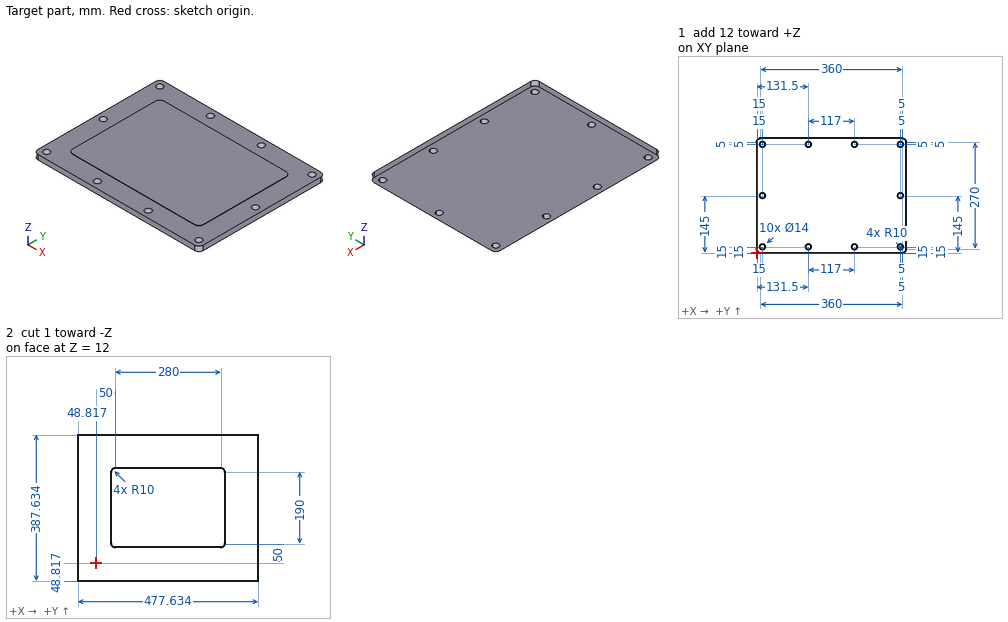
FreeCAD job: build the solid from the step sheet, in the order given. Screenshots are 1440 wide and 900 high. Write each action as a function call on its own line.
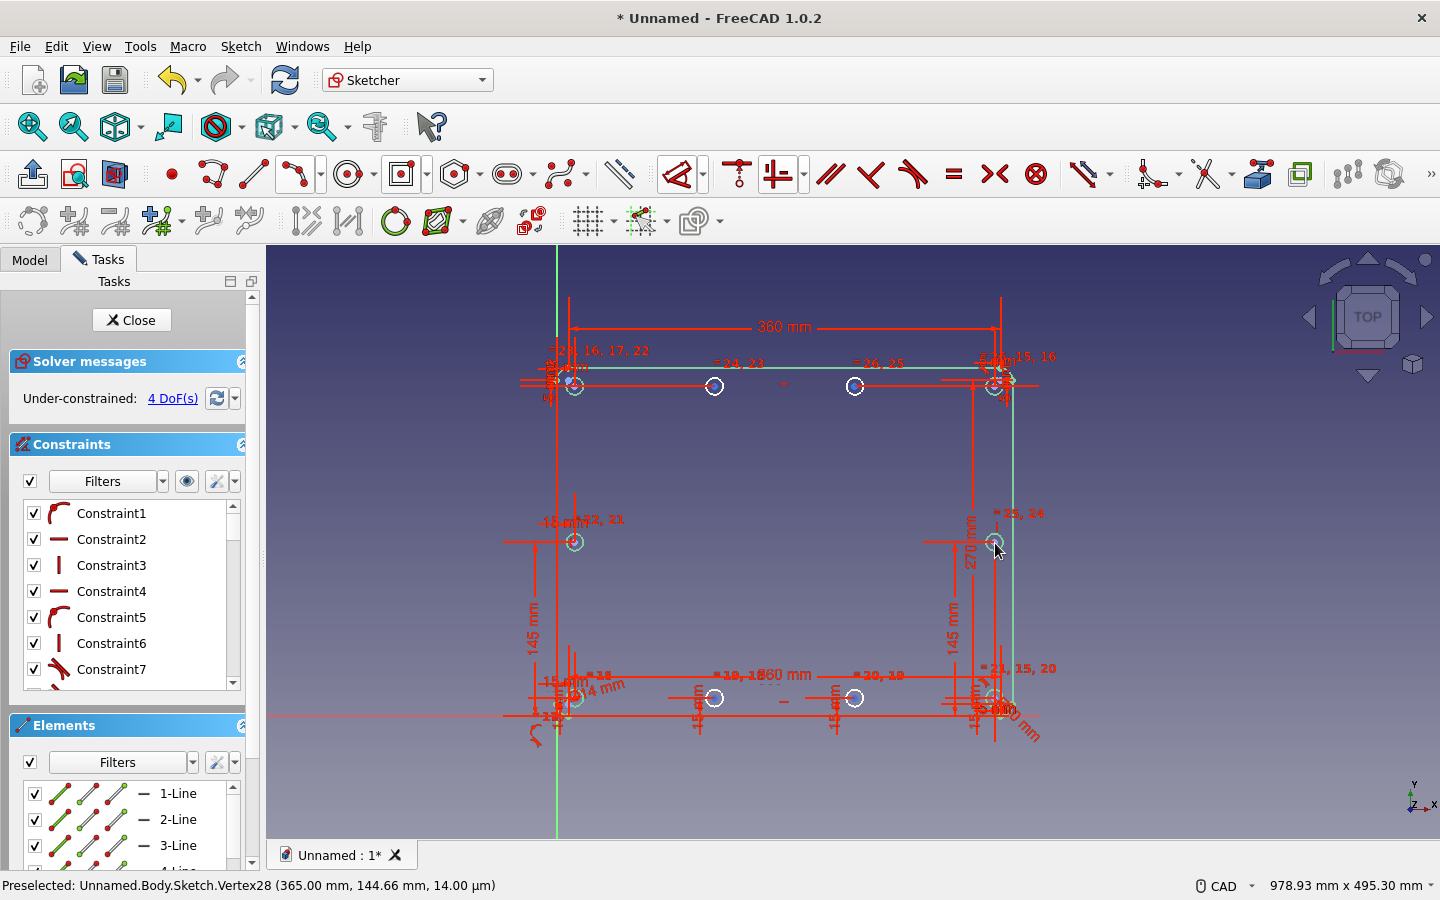
click(715, 698)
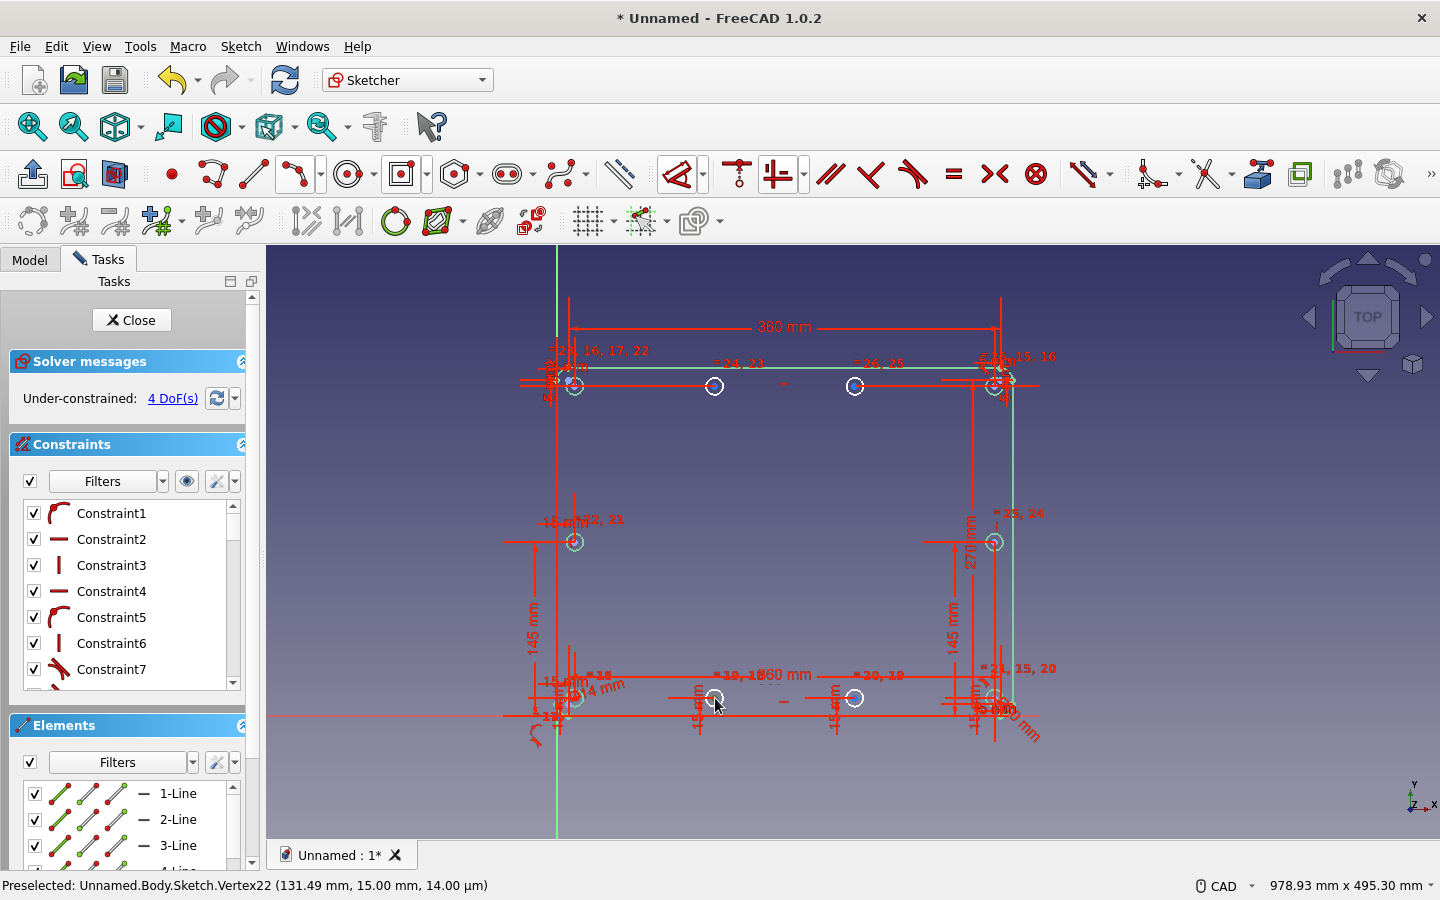
click(855, 698)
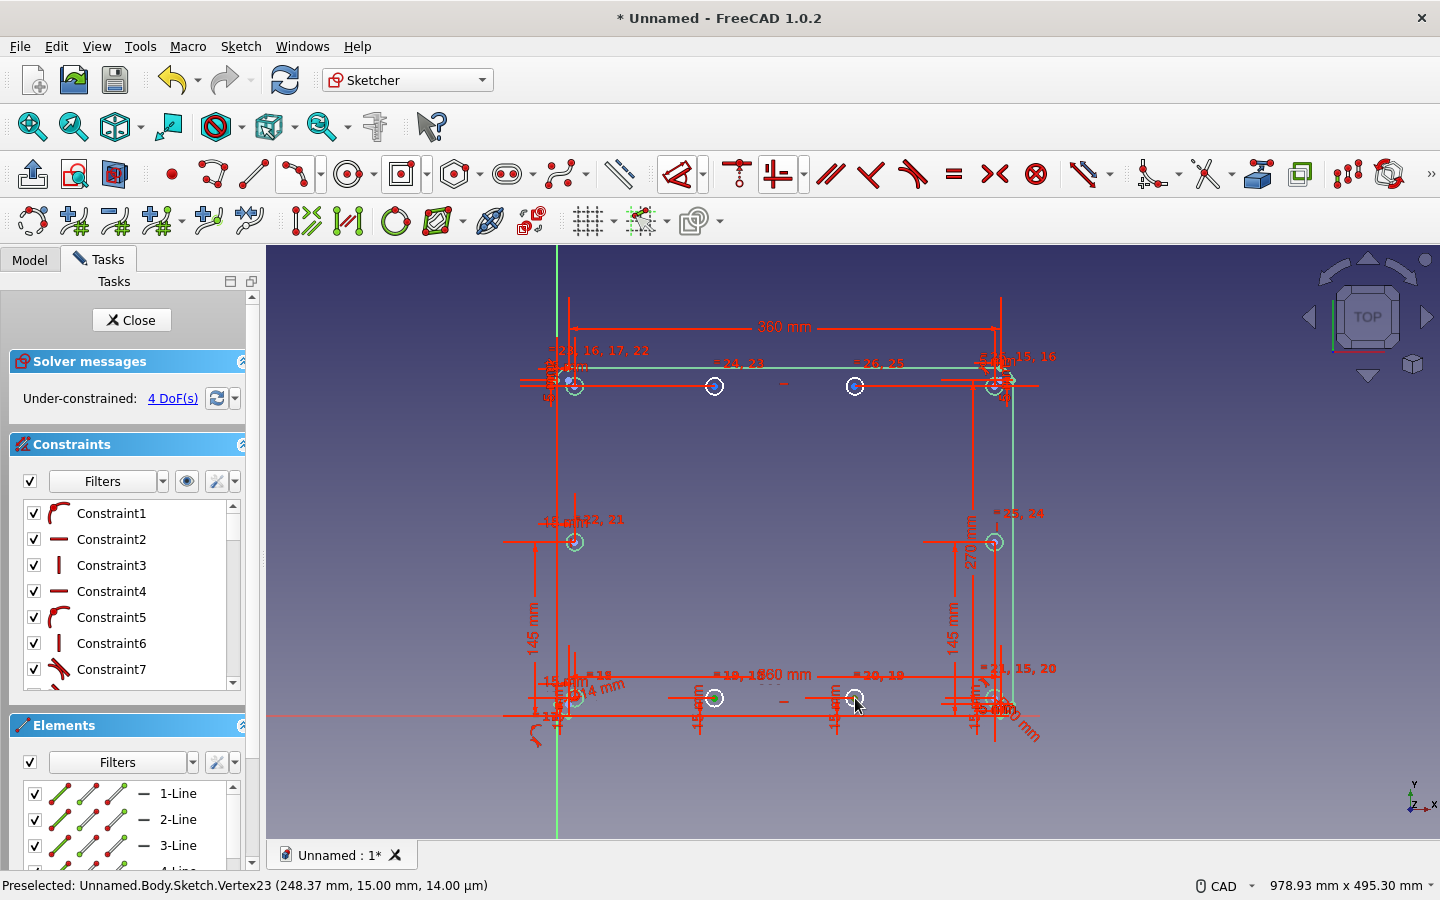
click(702, 174)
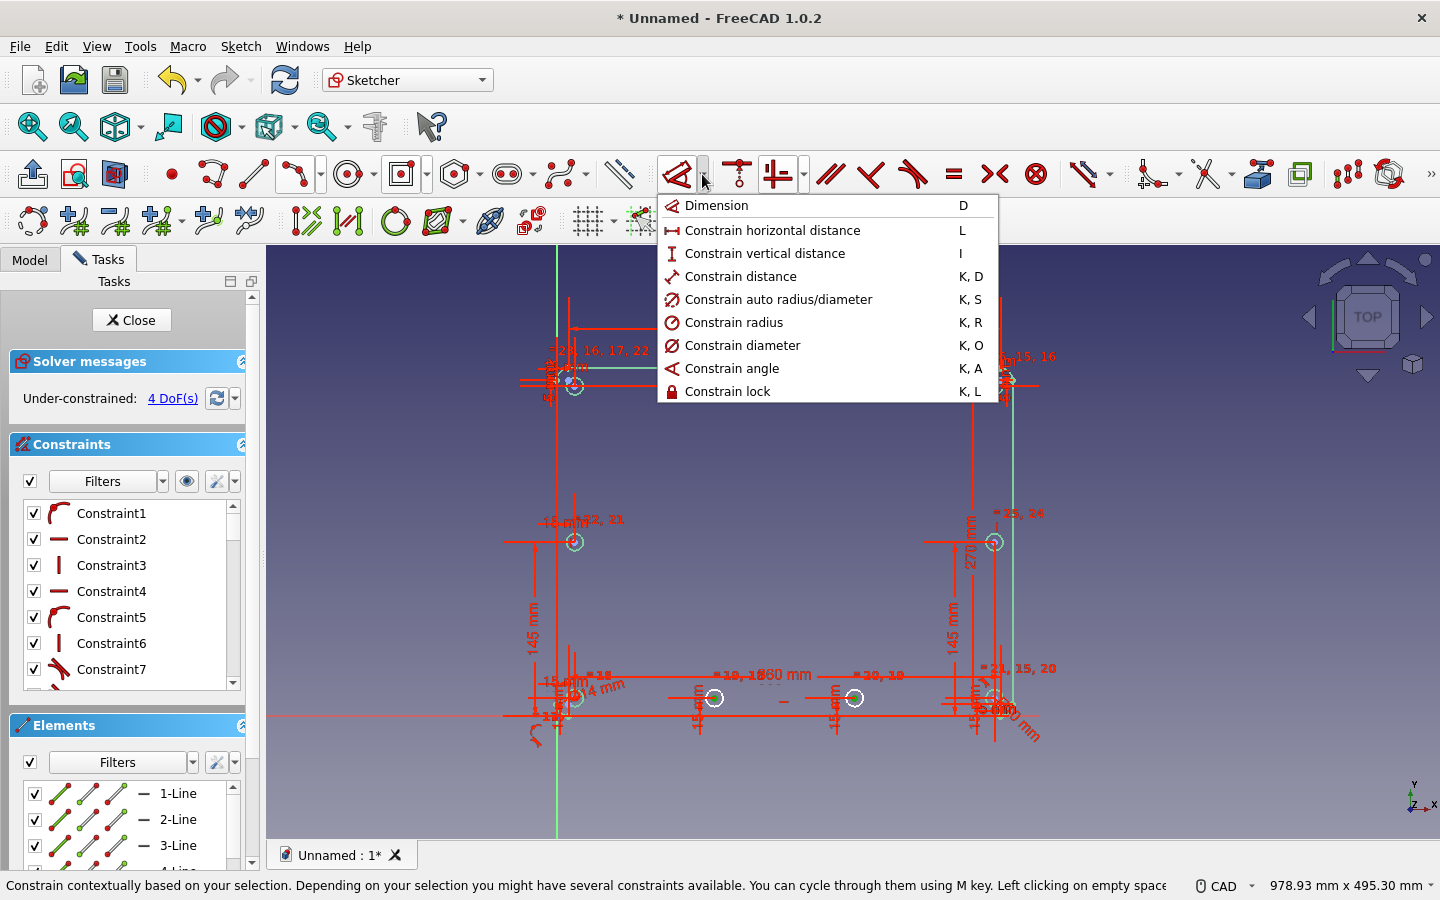
click(828, 230)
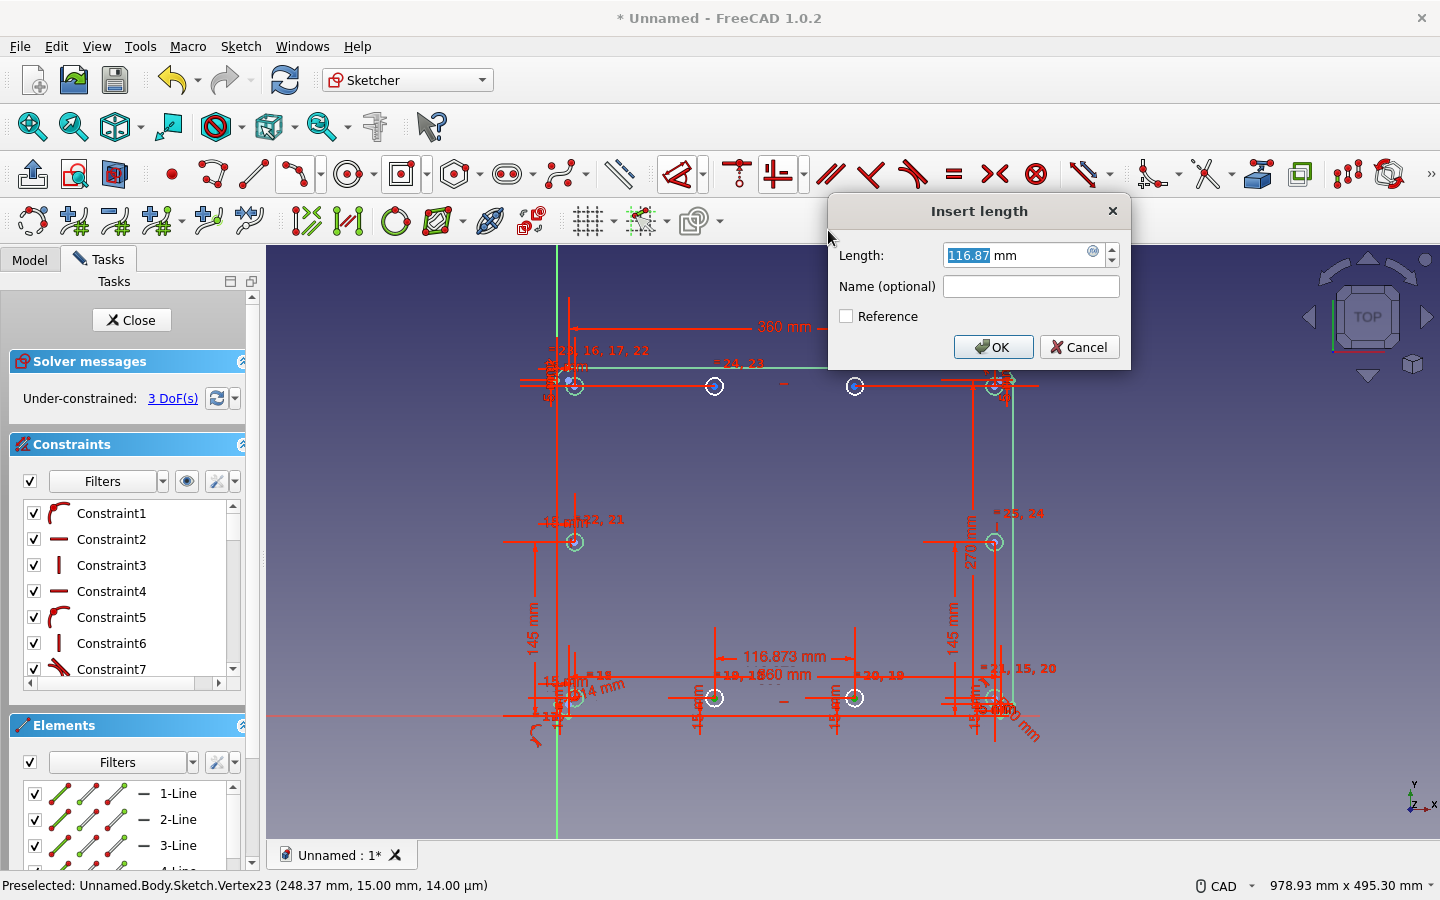
text(117)
key(Return)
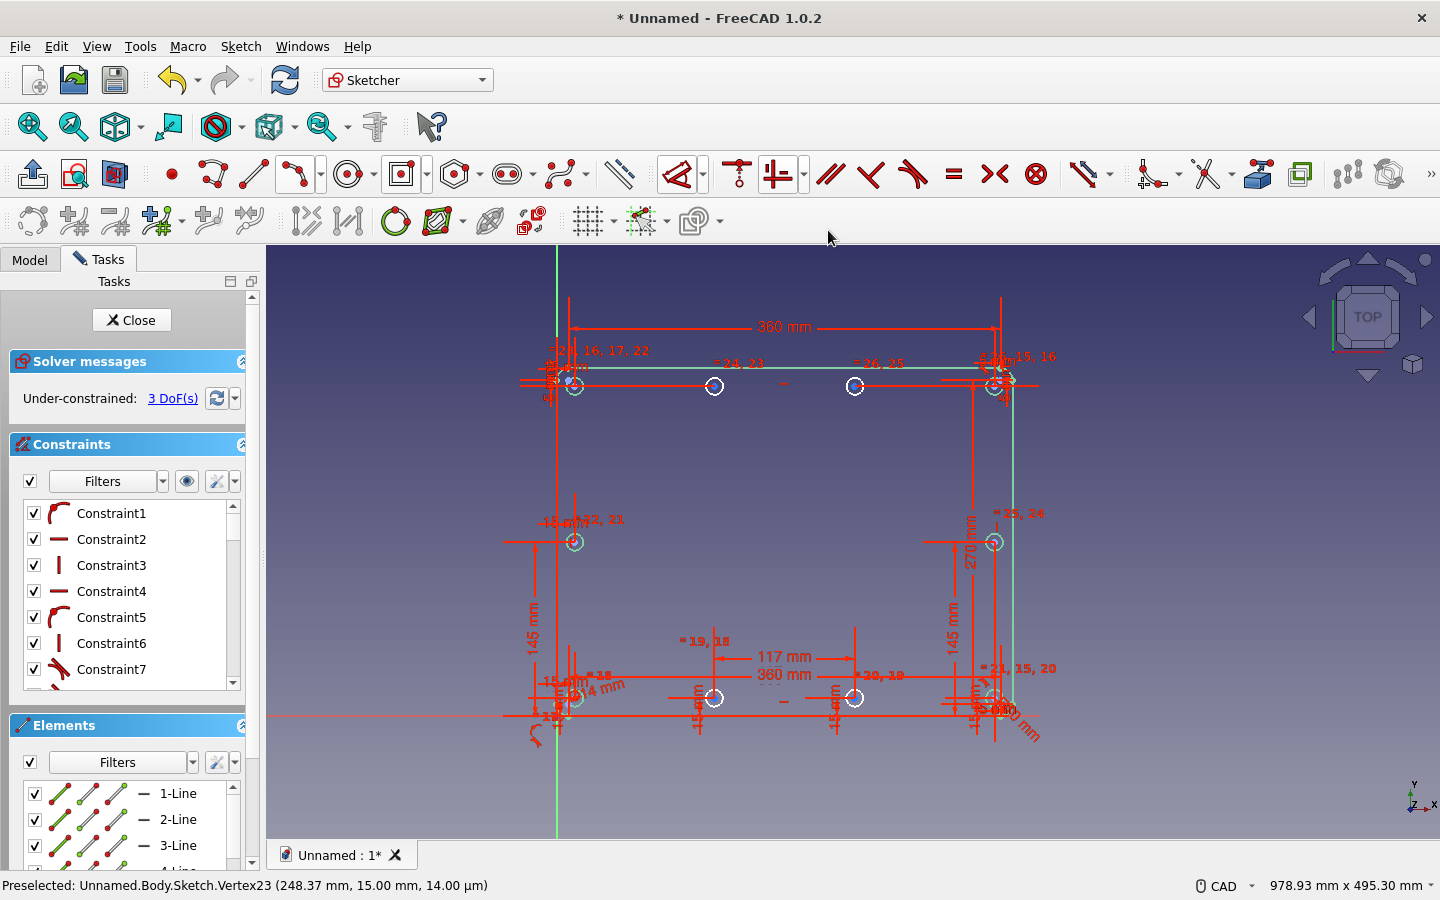
click(715, 386)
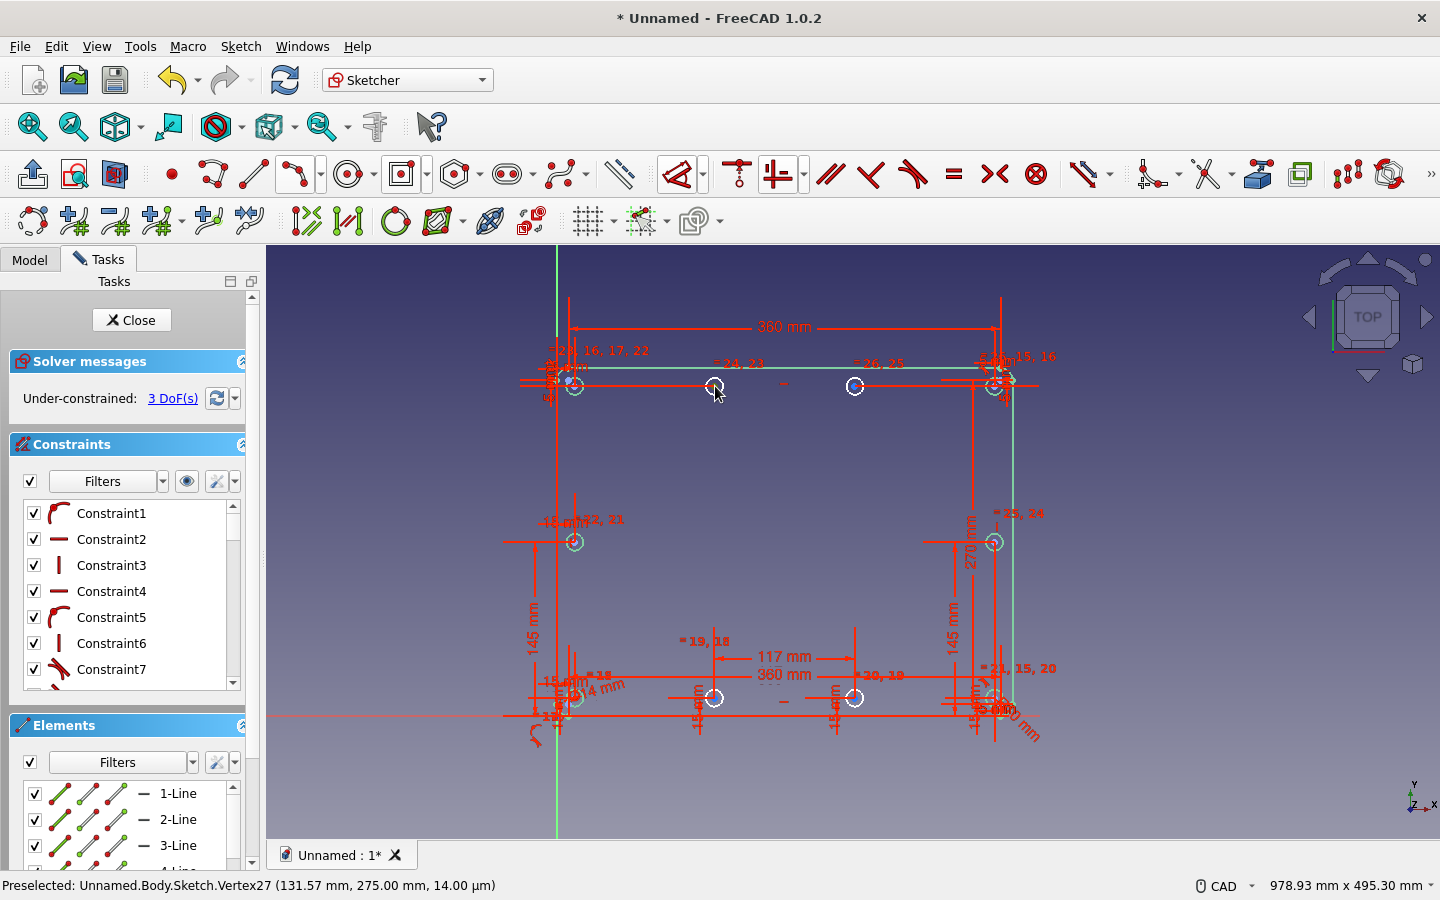
click(855, 386)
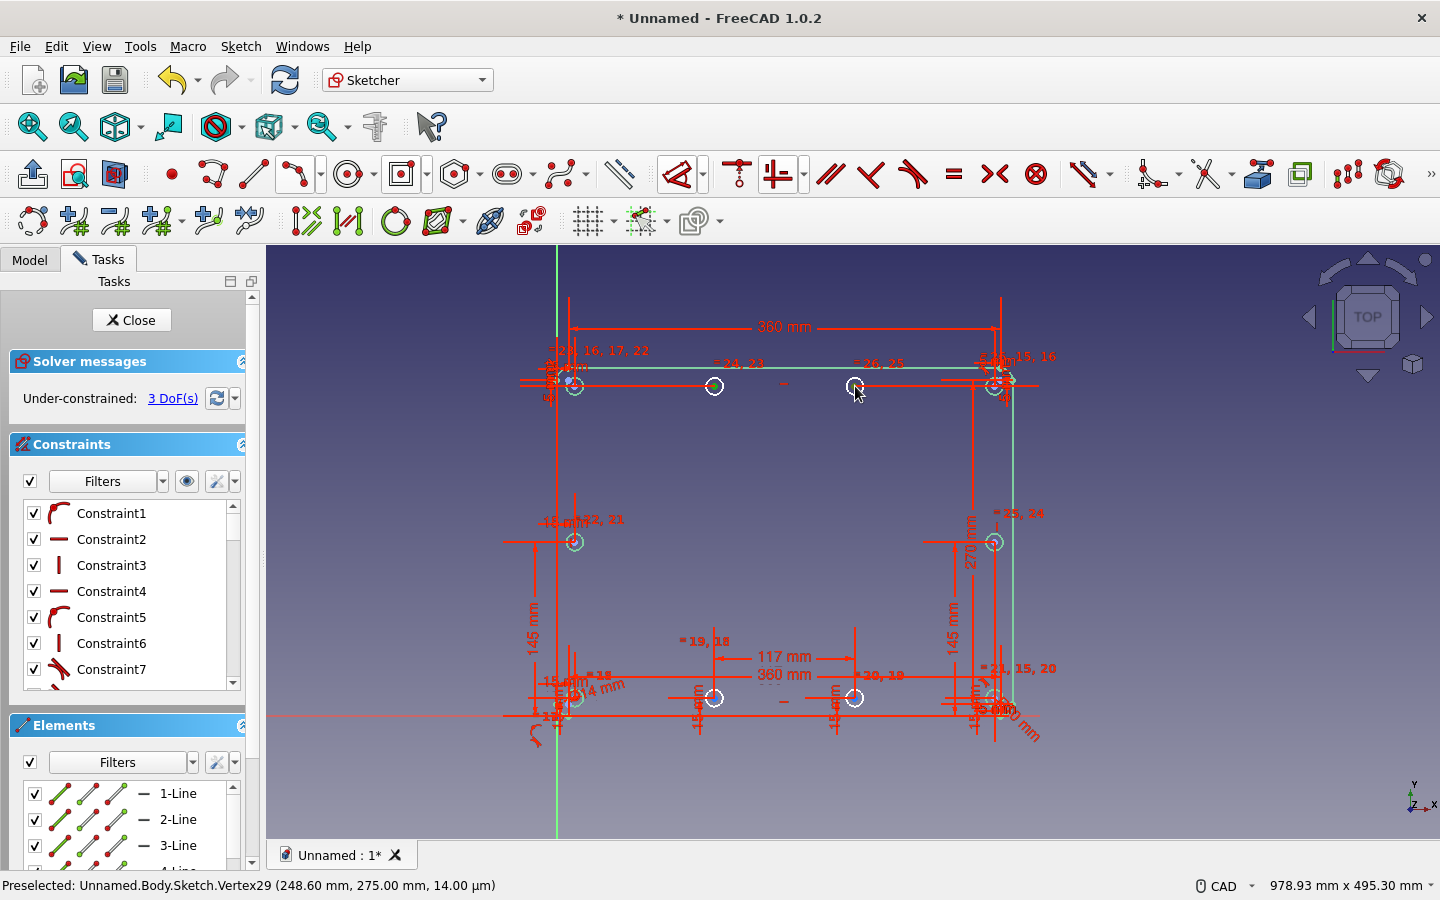
key(l)